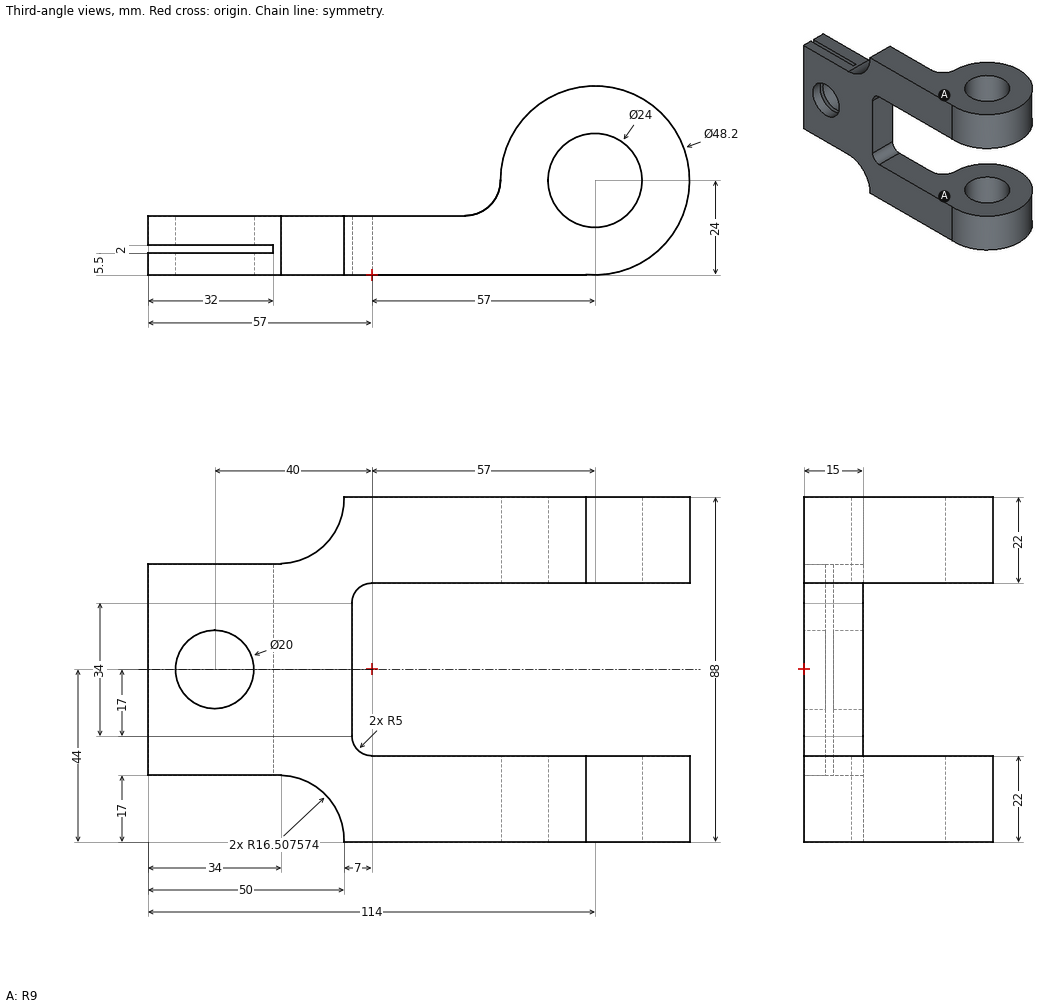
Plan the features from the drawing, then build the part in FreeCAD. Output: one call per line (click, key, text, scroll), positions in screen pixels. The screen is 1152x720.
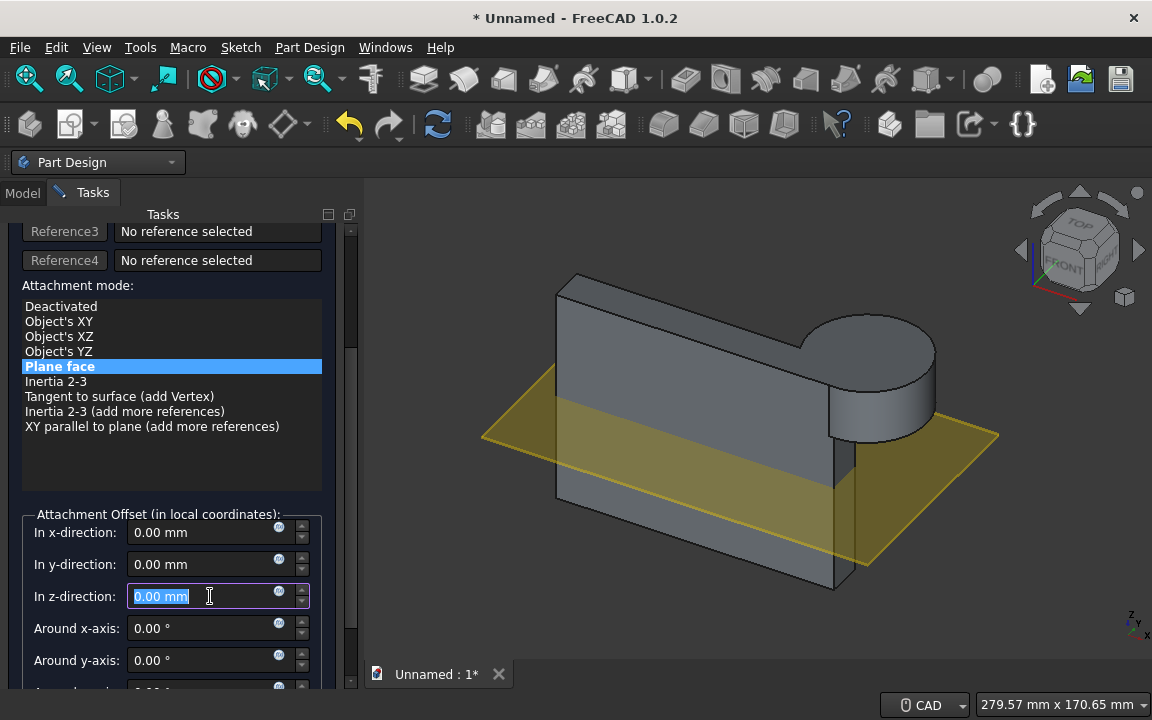
text(-22)
key(Tab)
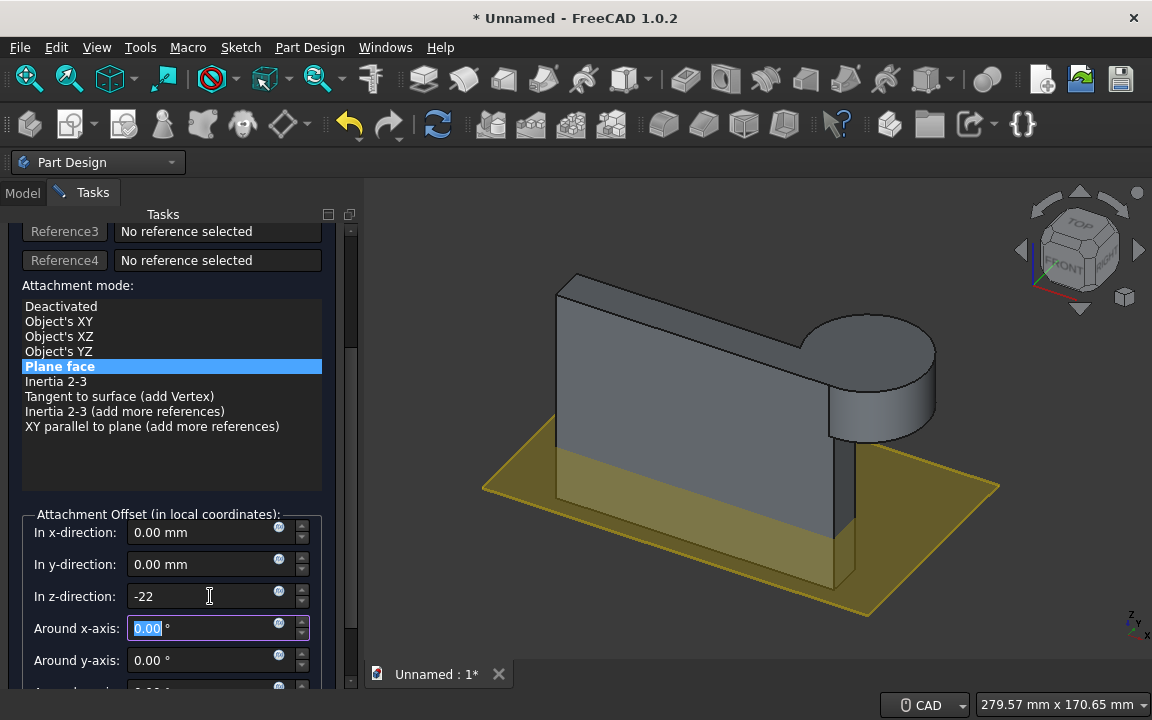
scroll(351, 456, up, 4)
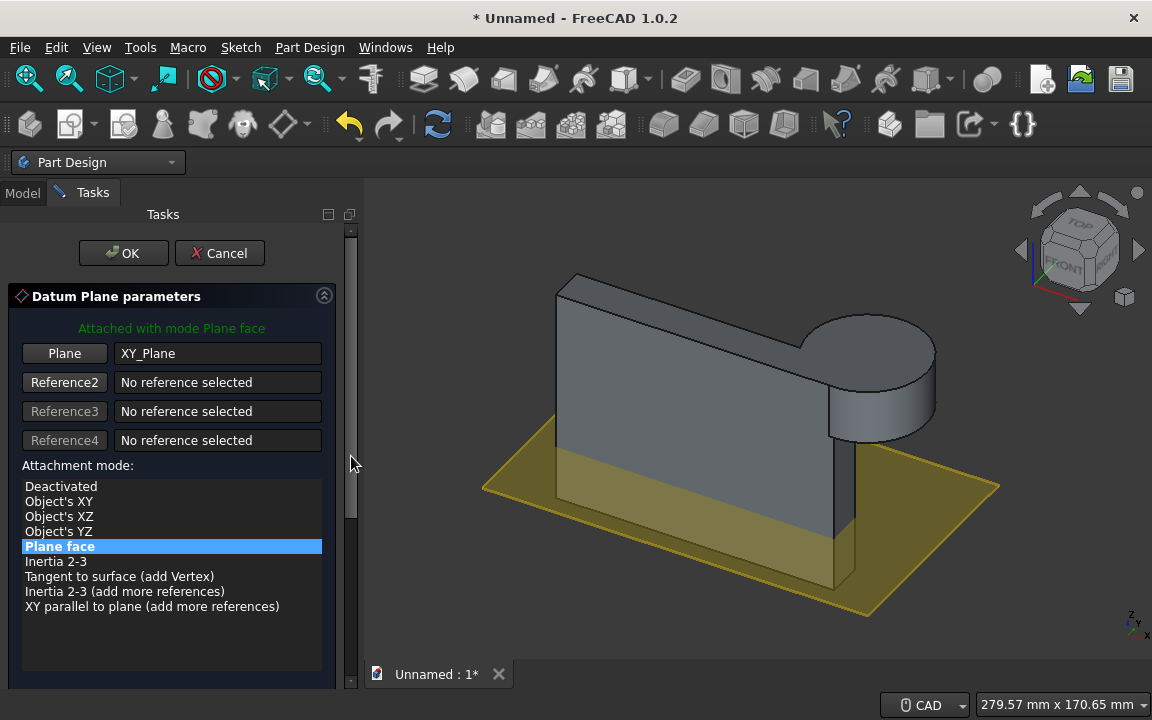
click(124, 253)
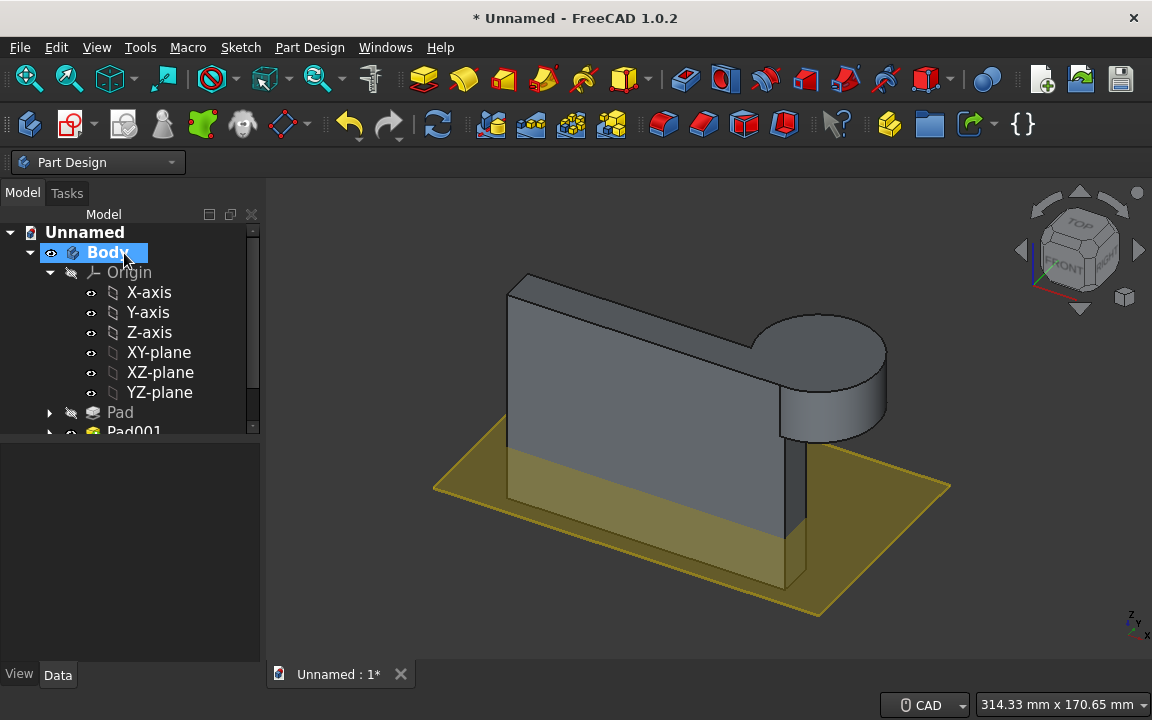
scroll(100, 328, down, 3)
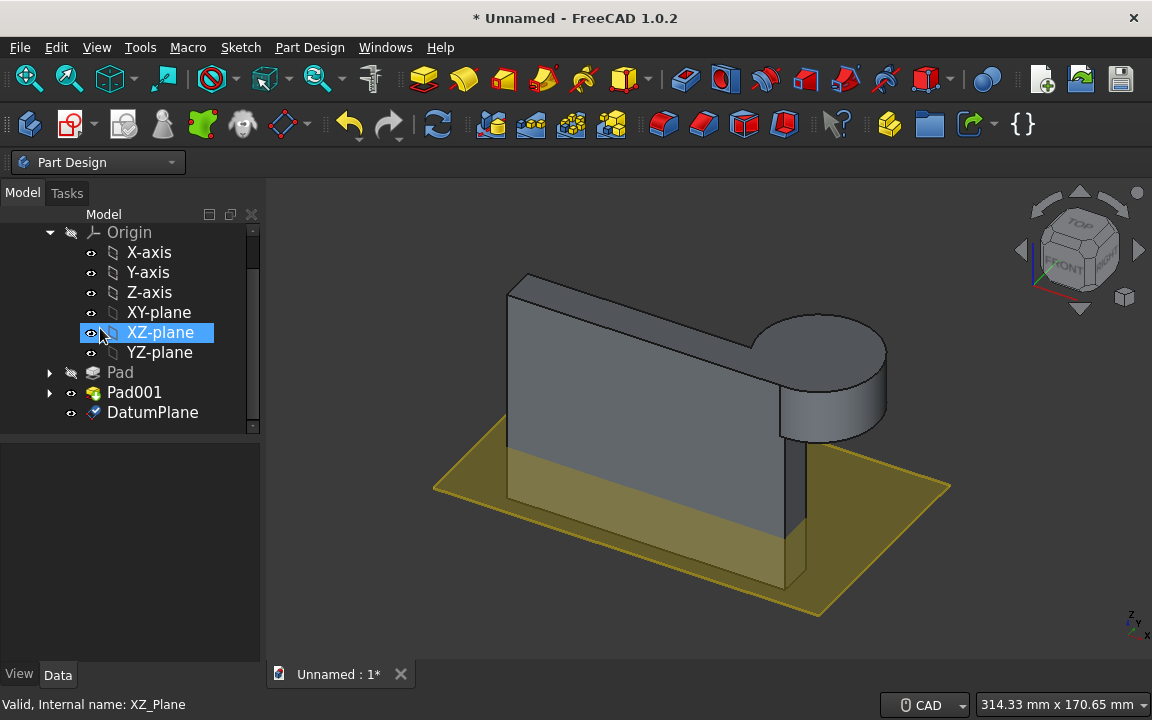
click(116, 413)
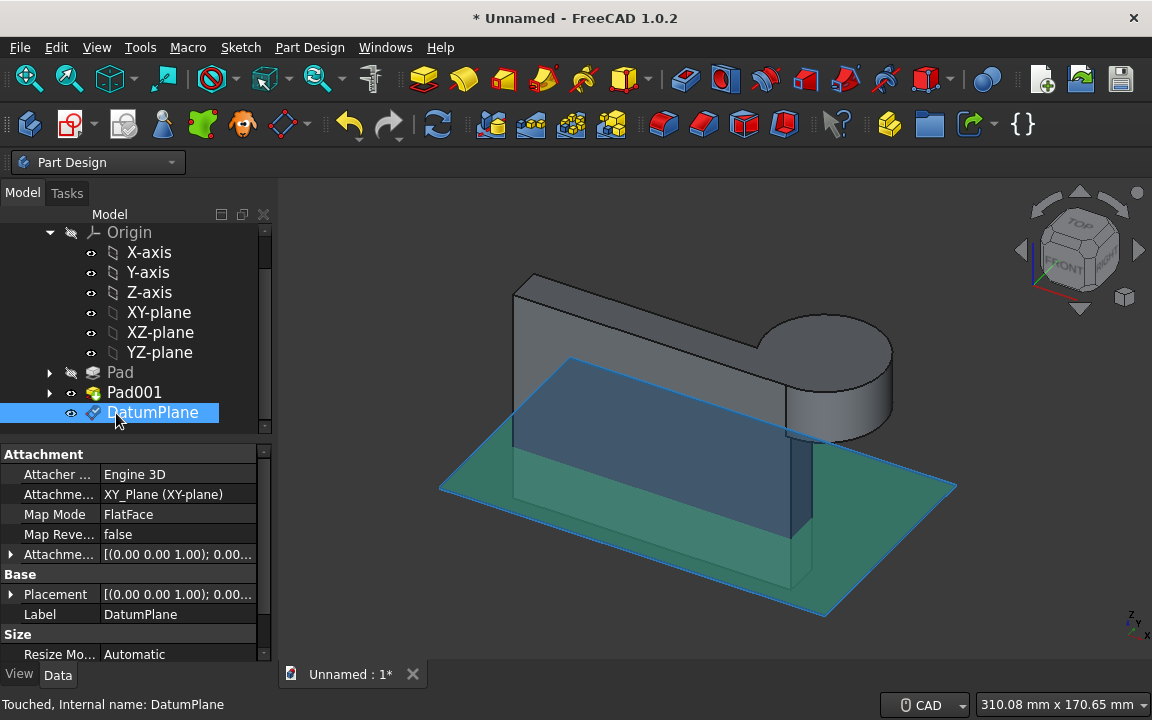
click(70, 124)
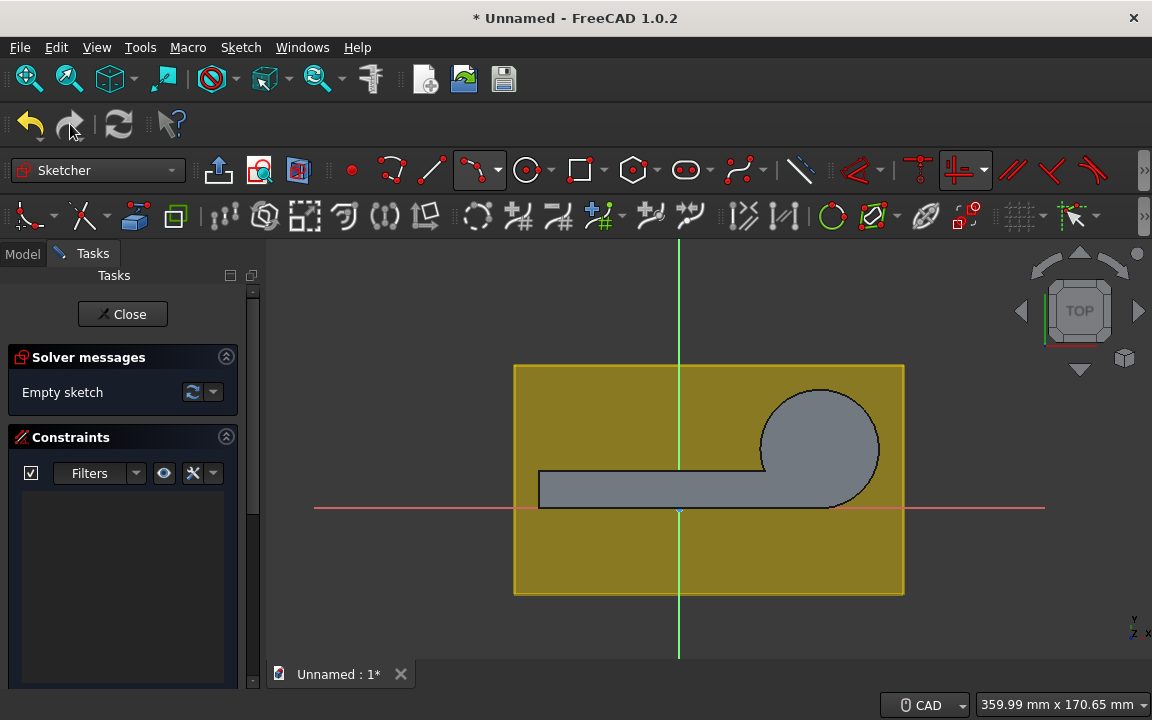
click(300, 170)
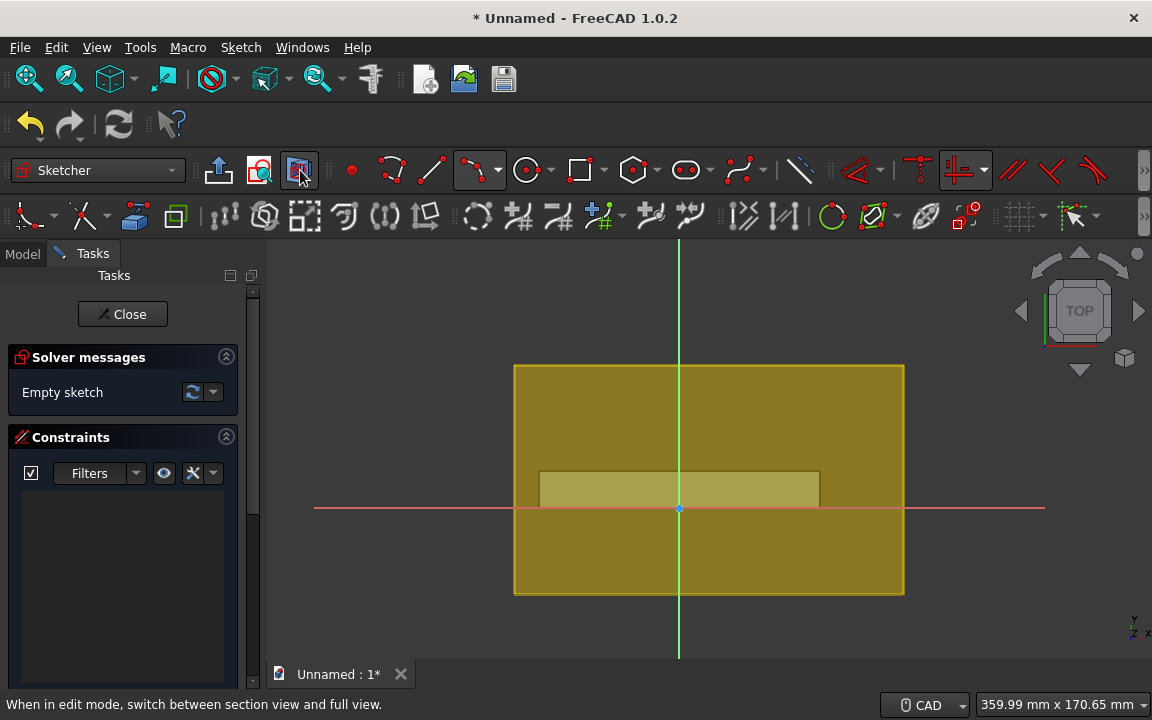
scroll(892, 449, up, 4)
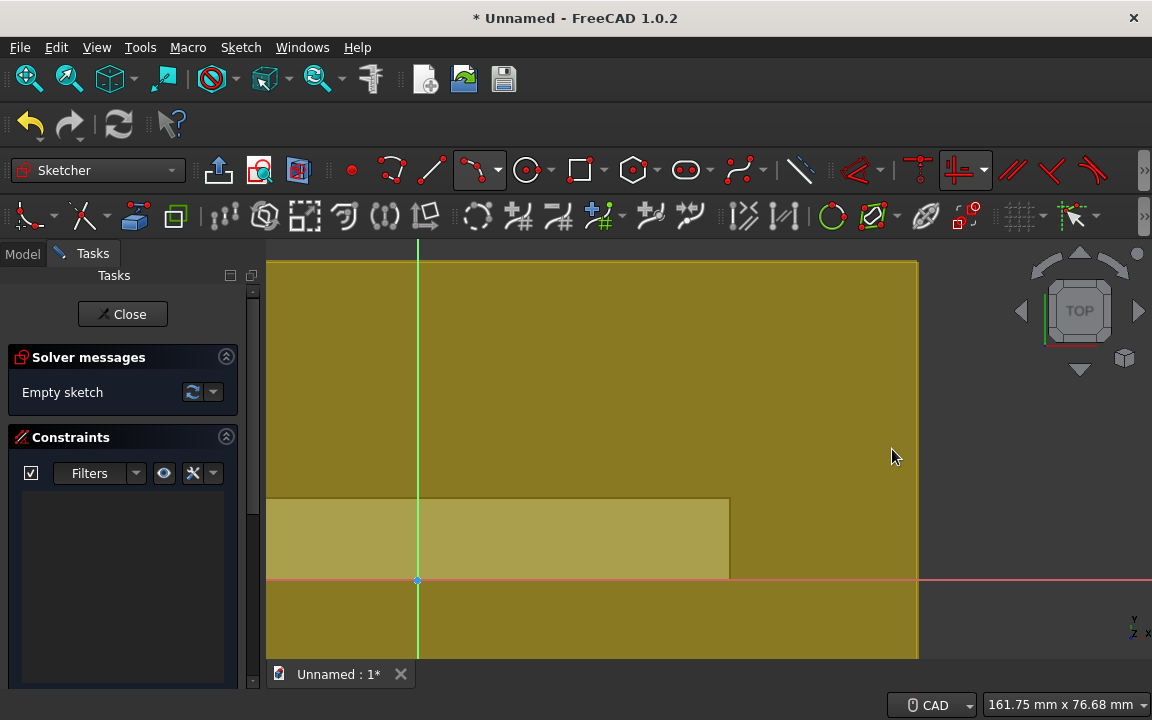
key(g)
key(c)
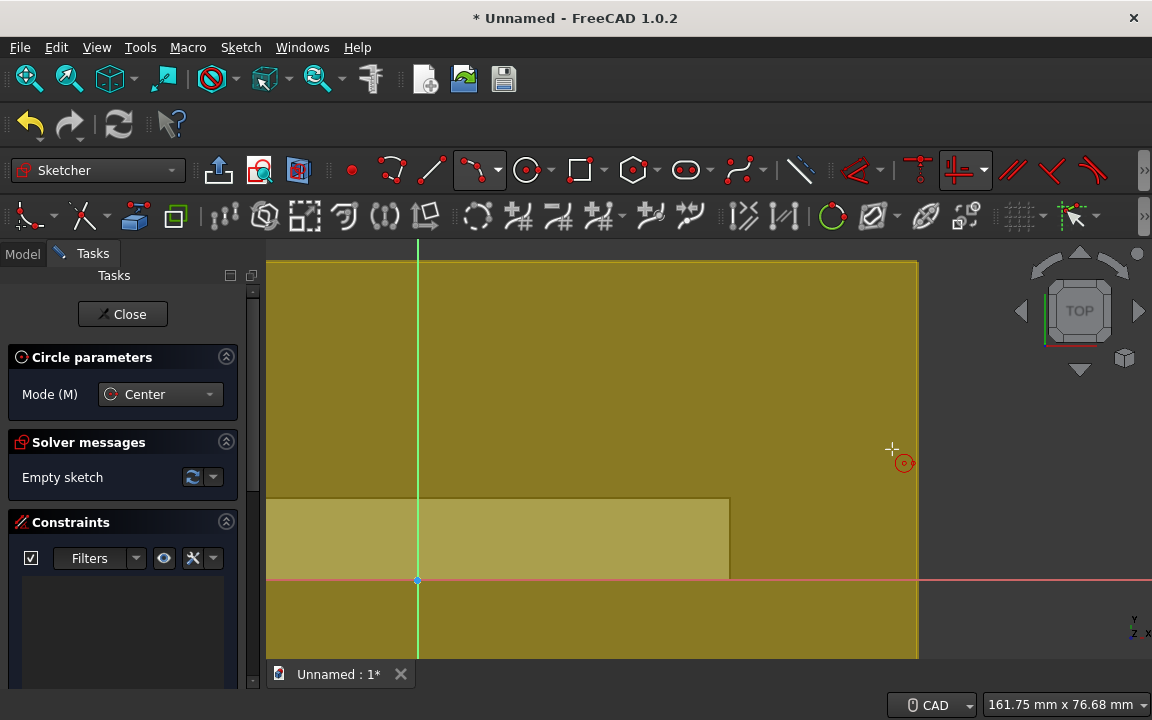
click(730, 449)
move(824, 355)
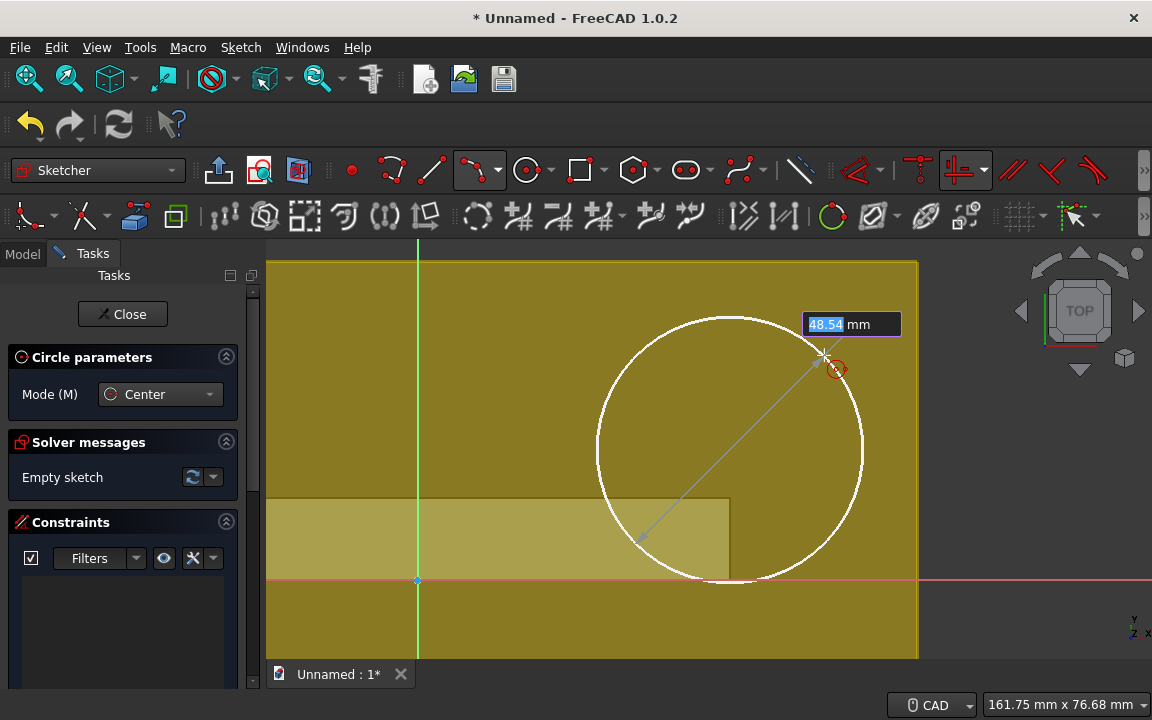
text(48.2)
key(Return)
key(Escape)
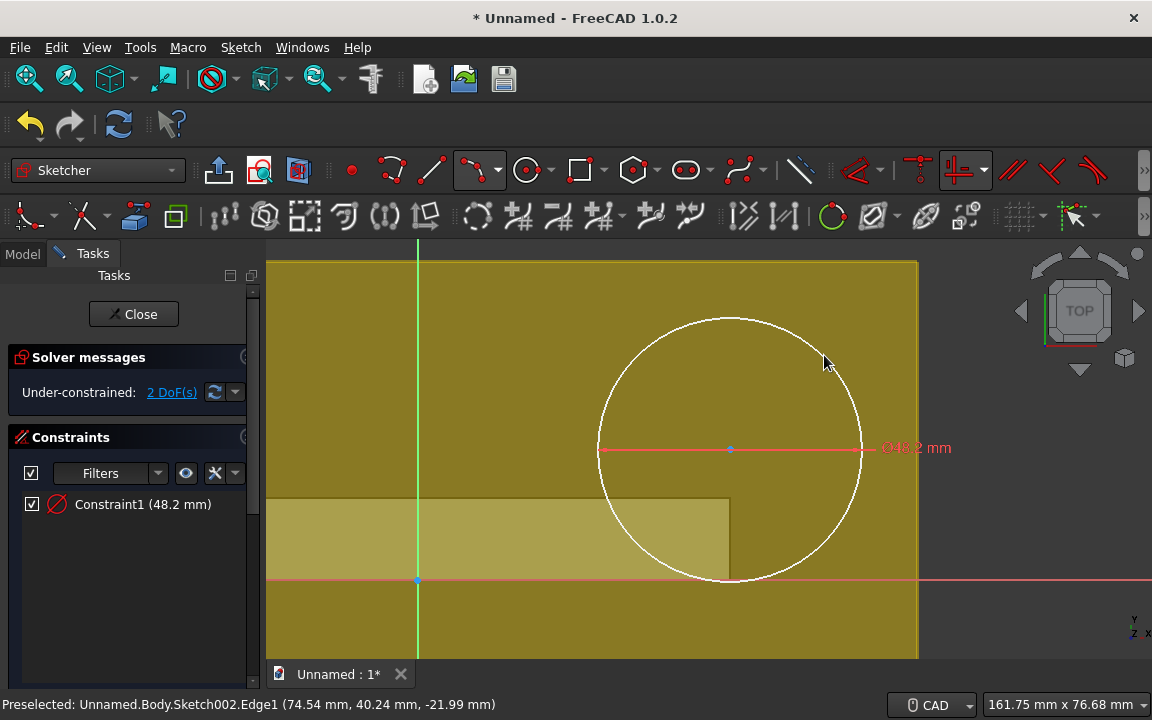
key(d)